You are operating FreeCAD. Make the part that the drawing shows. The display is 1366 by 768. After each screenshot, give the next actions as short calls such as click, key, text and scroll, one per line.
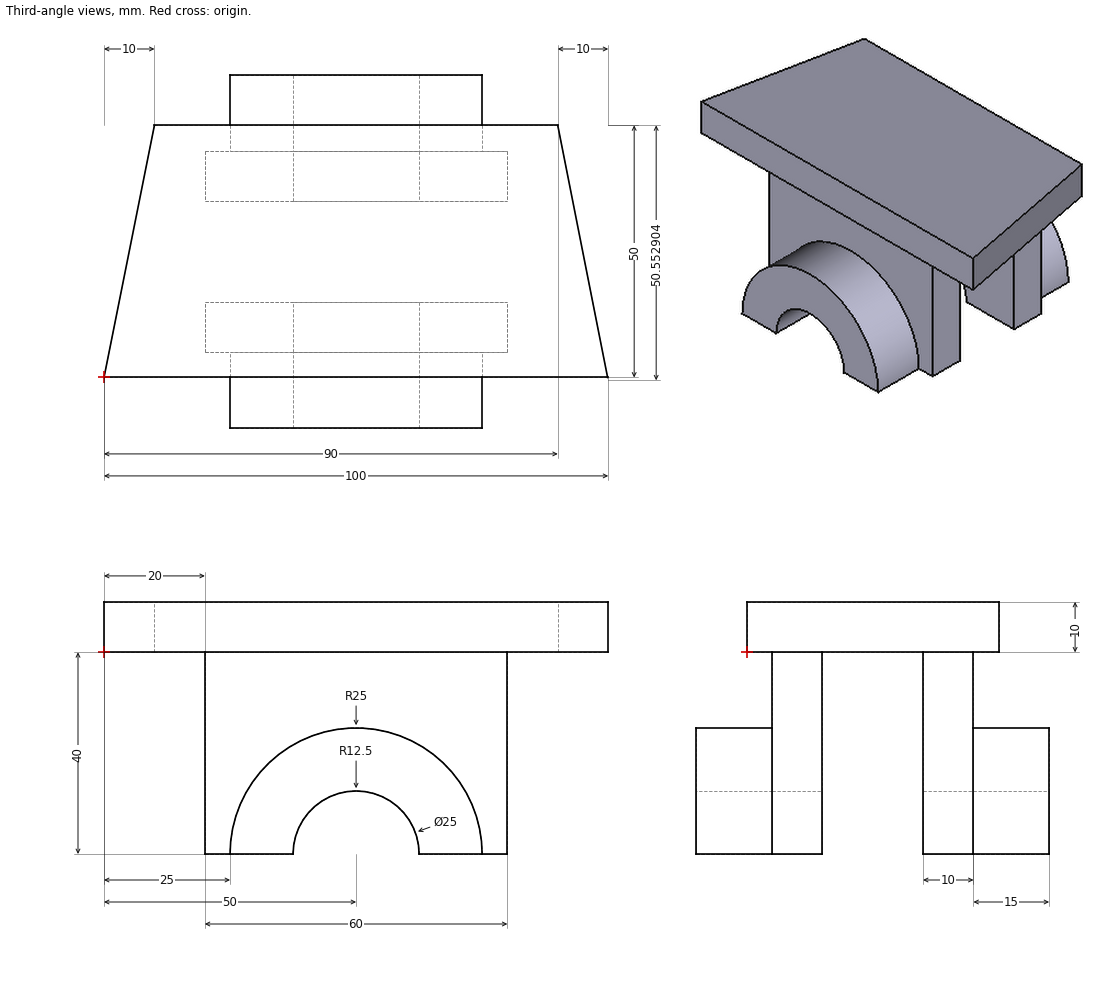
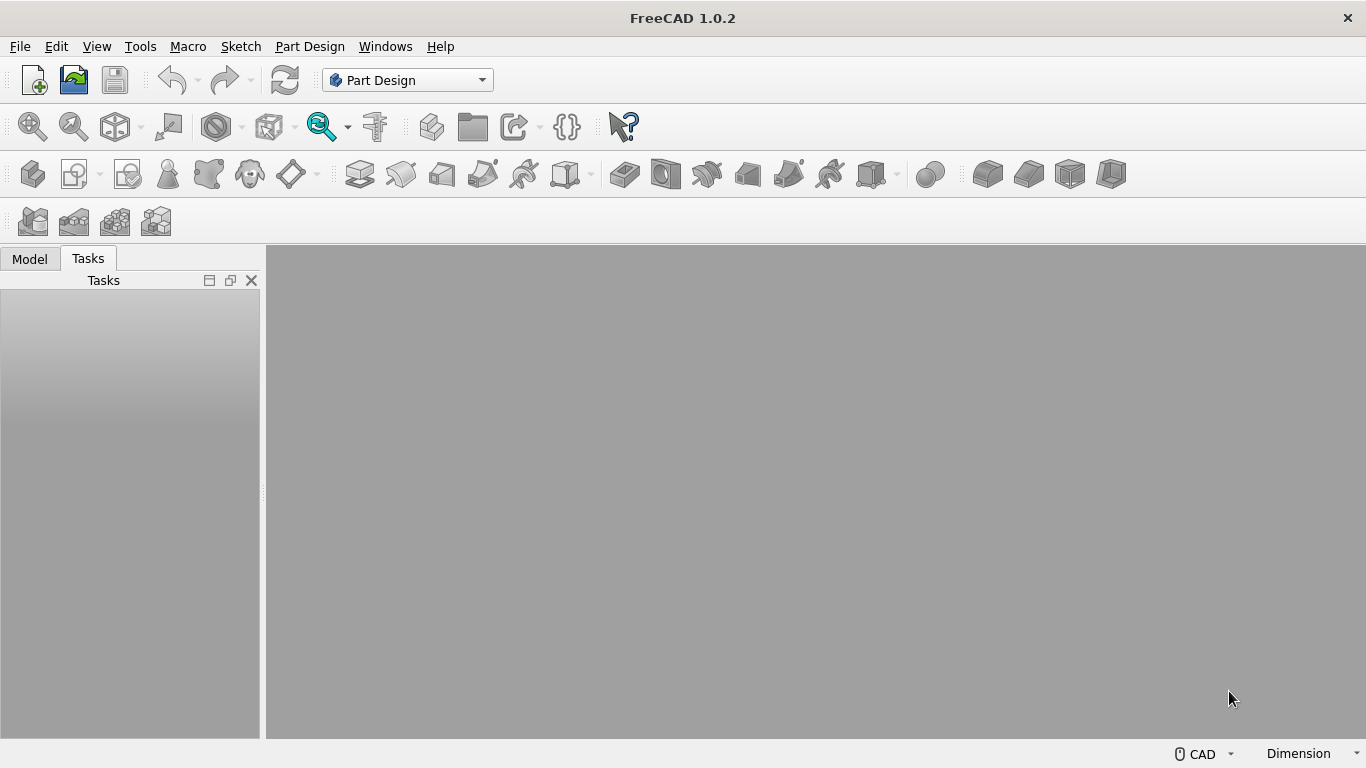
key(ctrl+n)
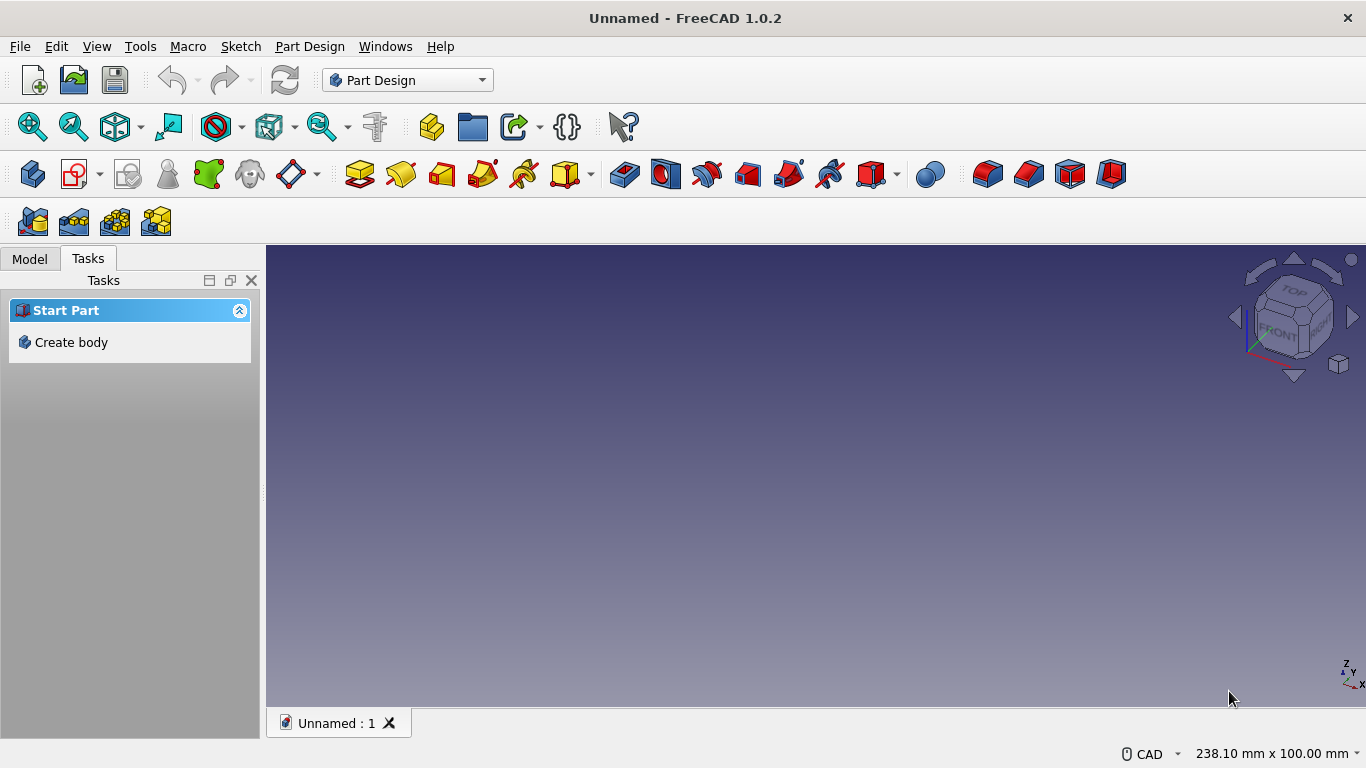
click(74, 174)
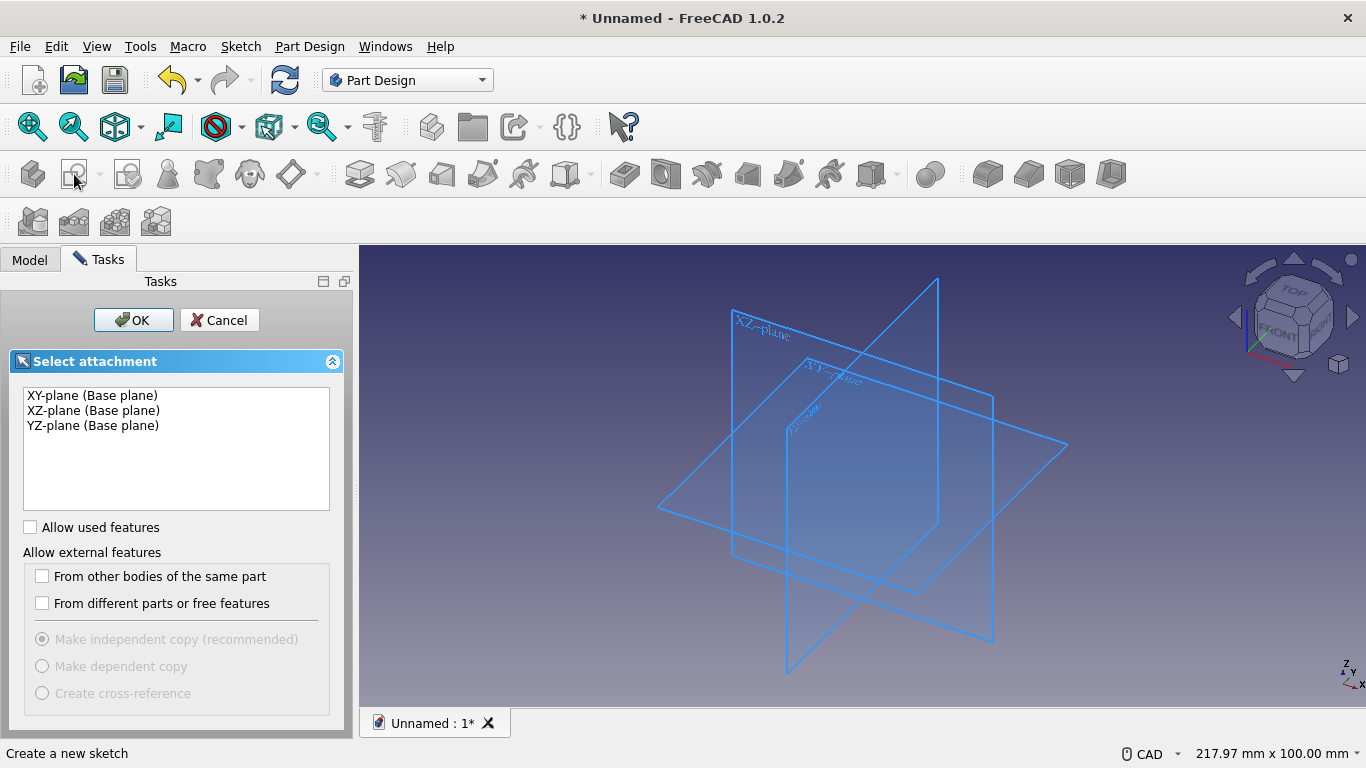
click(84, 396)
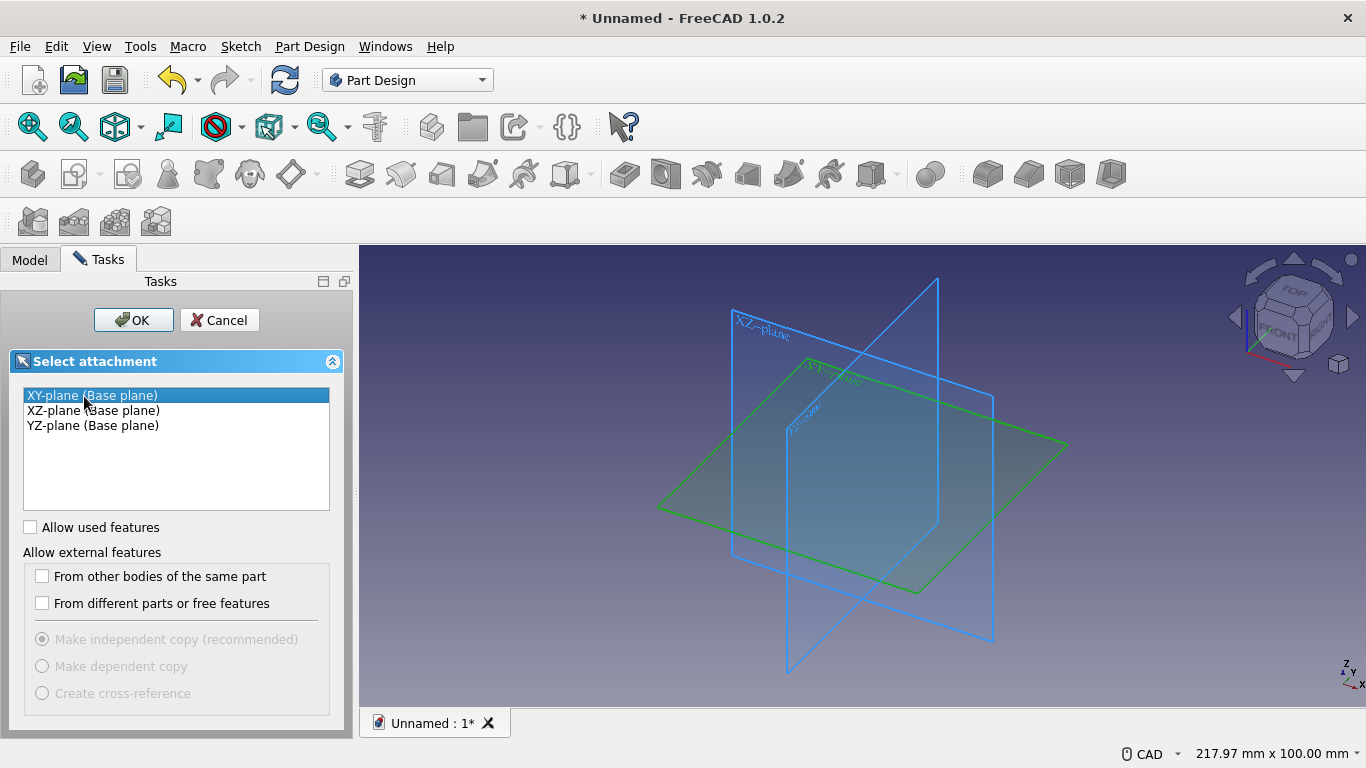
click(134, 320)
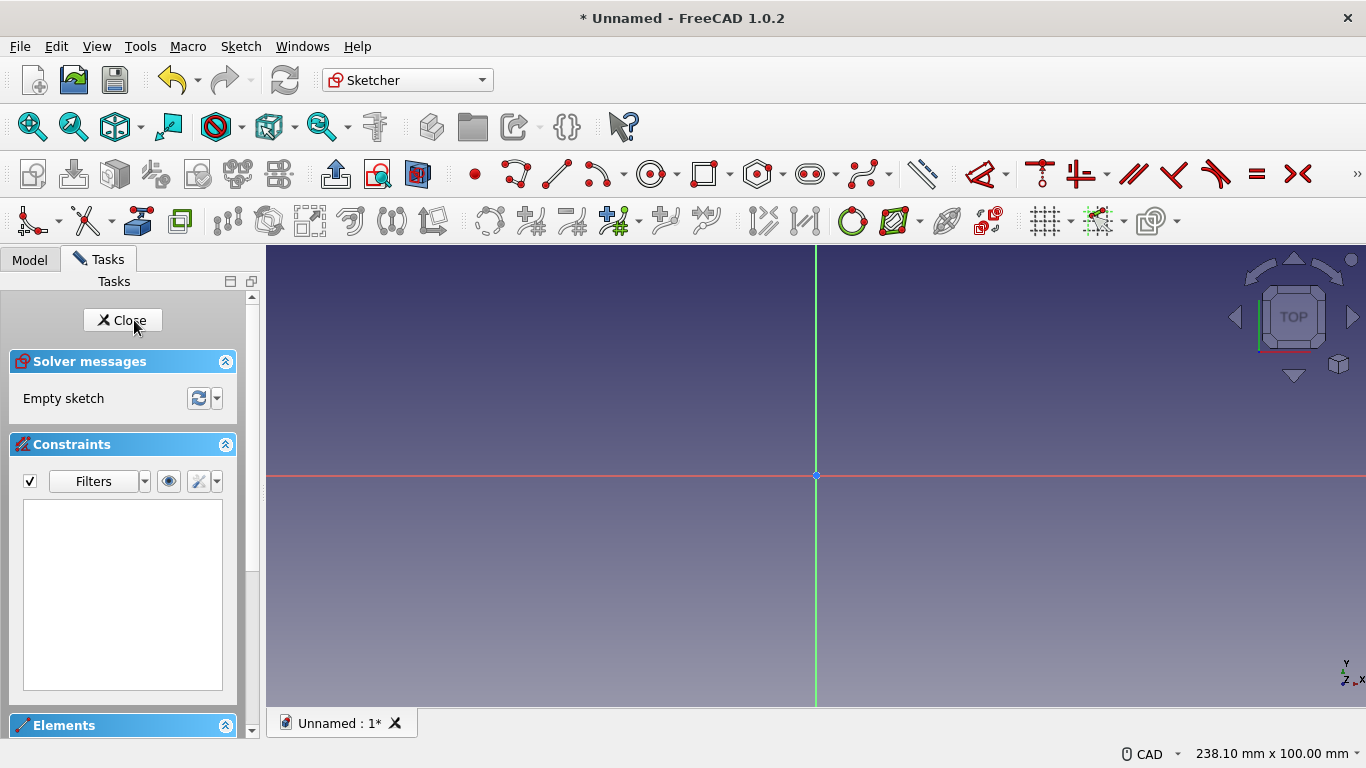
scroll(294, 679, down, 1)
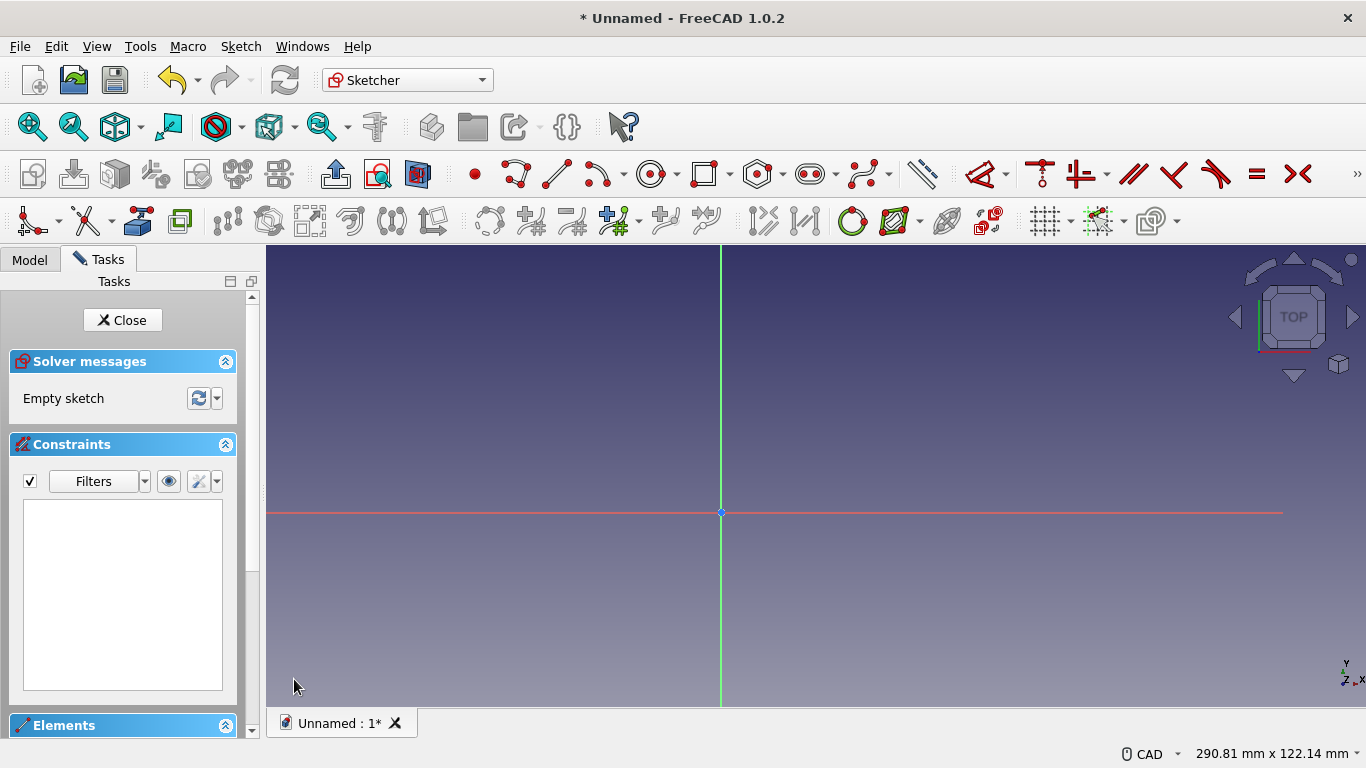
scroll(1201, 301, up, 2)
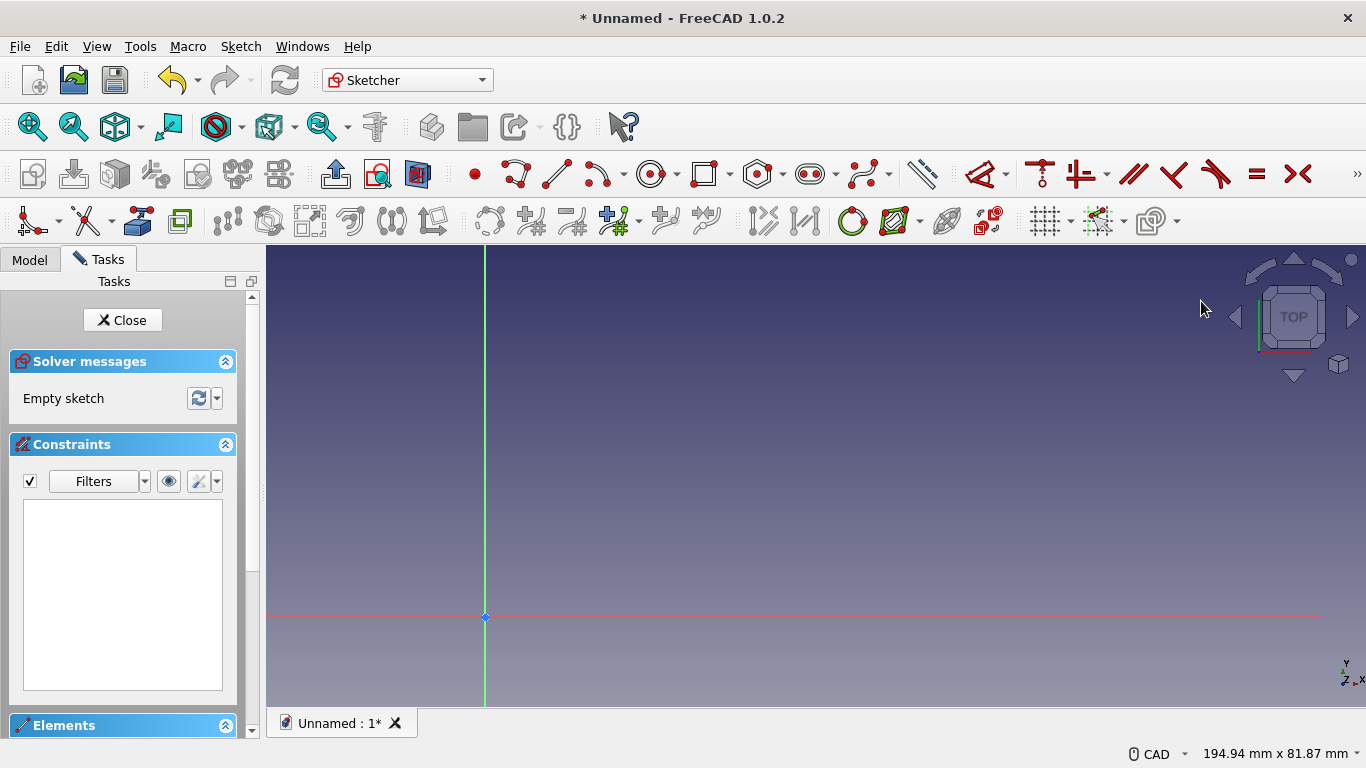
click(704, 174)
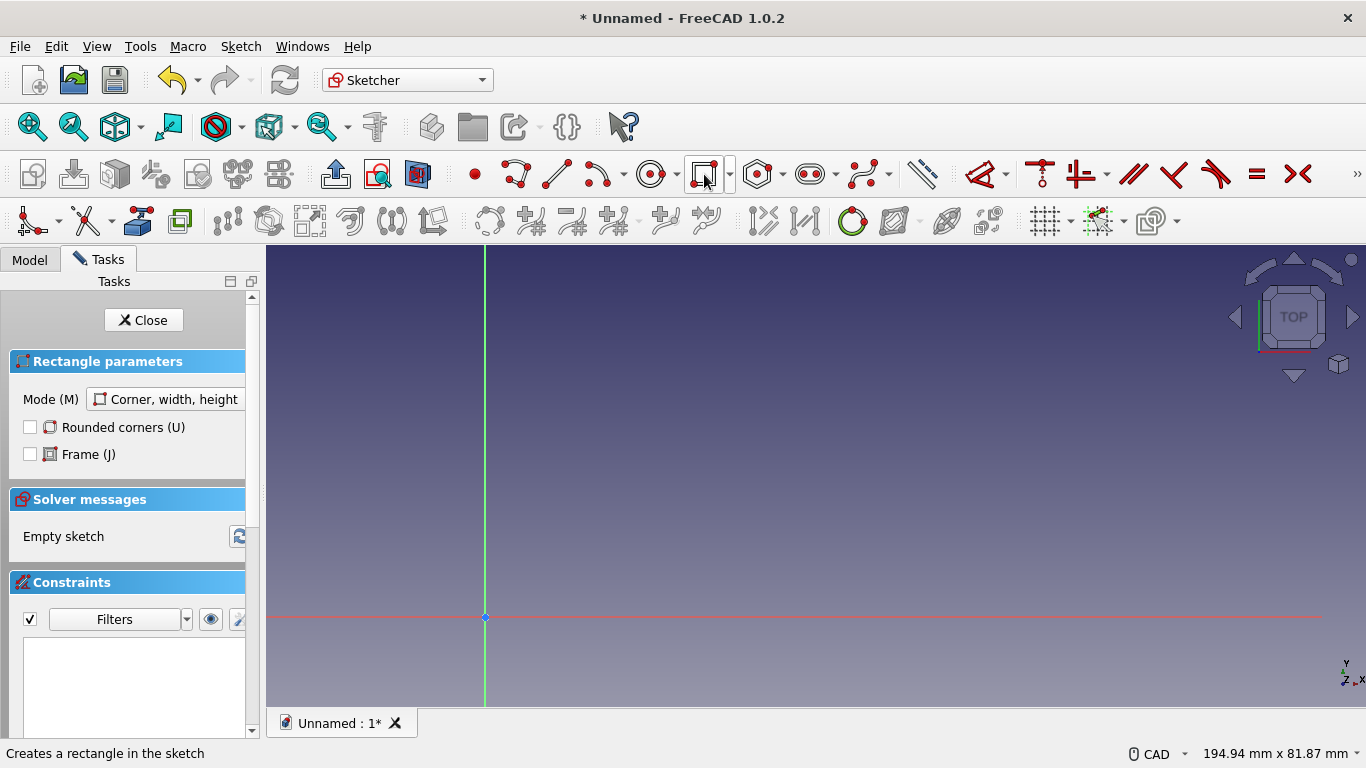
click(485, 617)
click(1049, 335)
key(Escape)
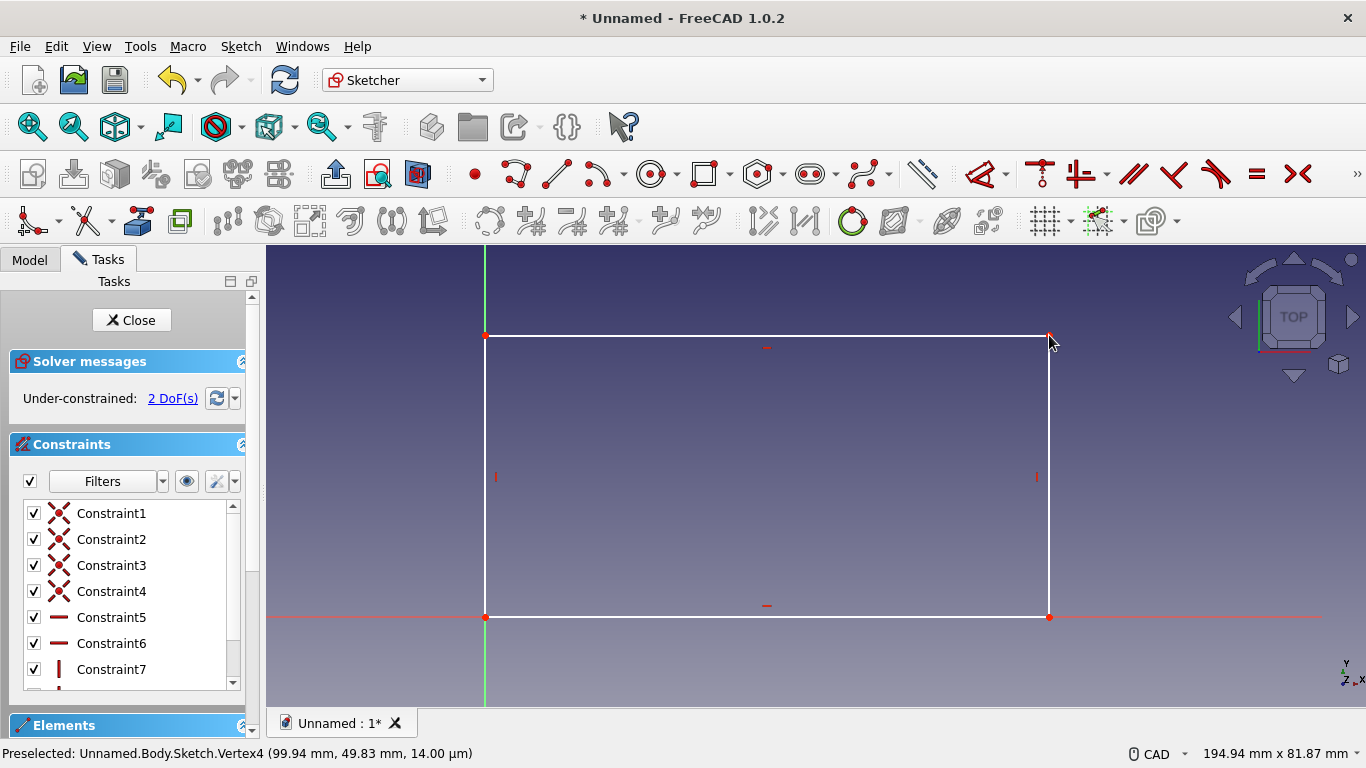
key(d)